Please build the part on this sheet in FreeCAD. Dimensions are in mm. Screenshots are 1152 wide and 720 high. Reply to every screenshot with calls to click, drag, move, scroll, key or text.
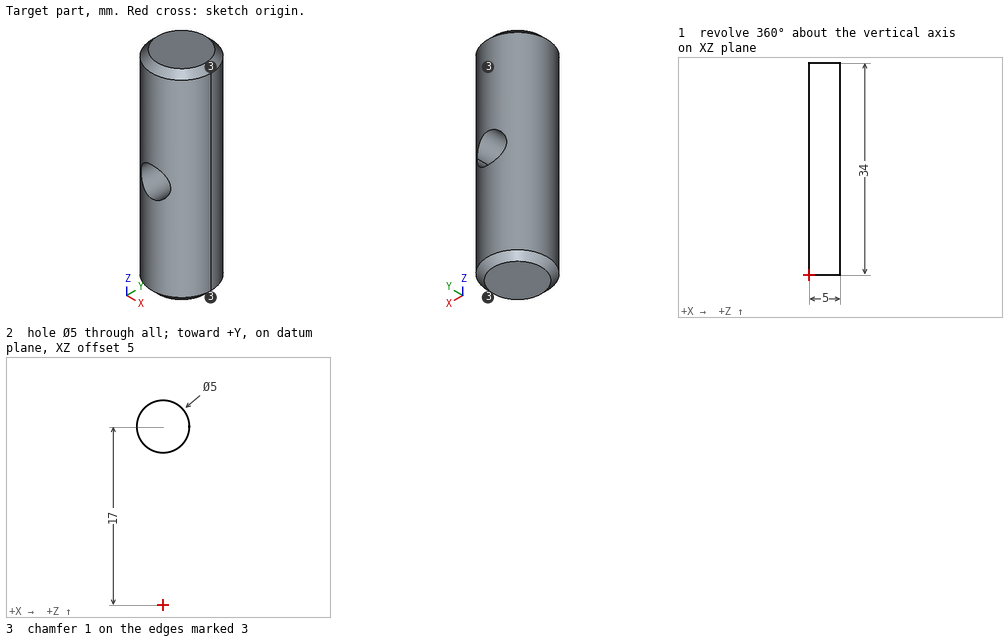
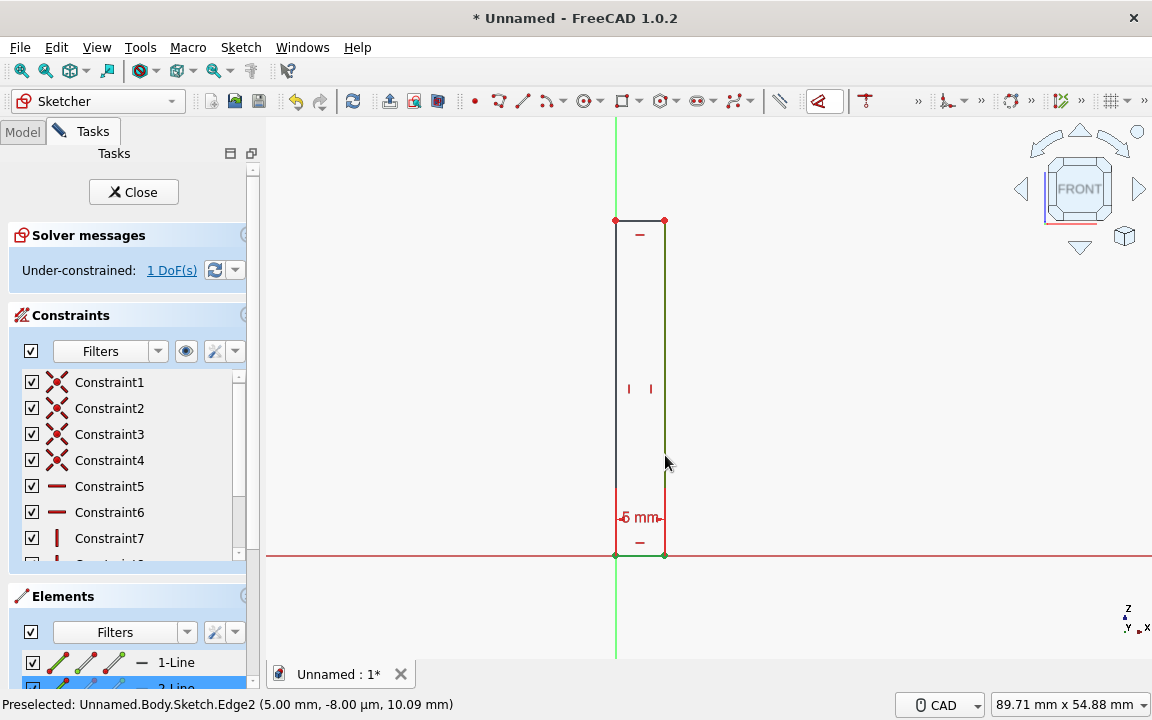
key(i)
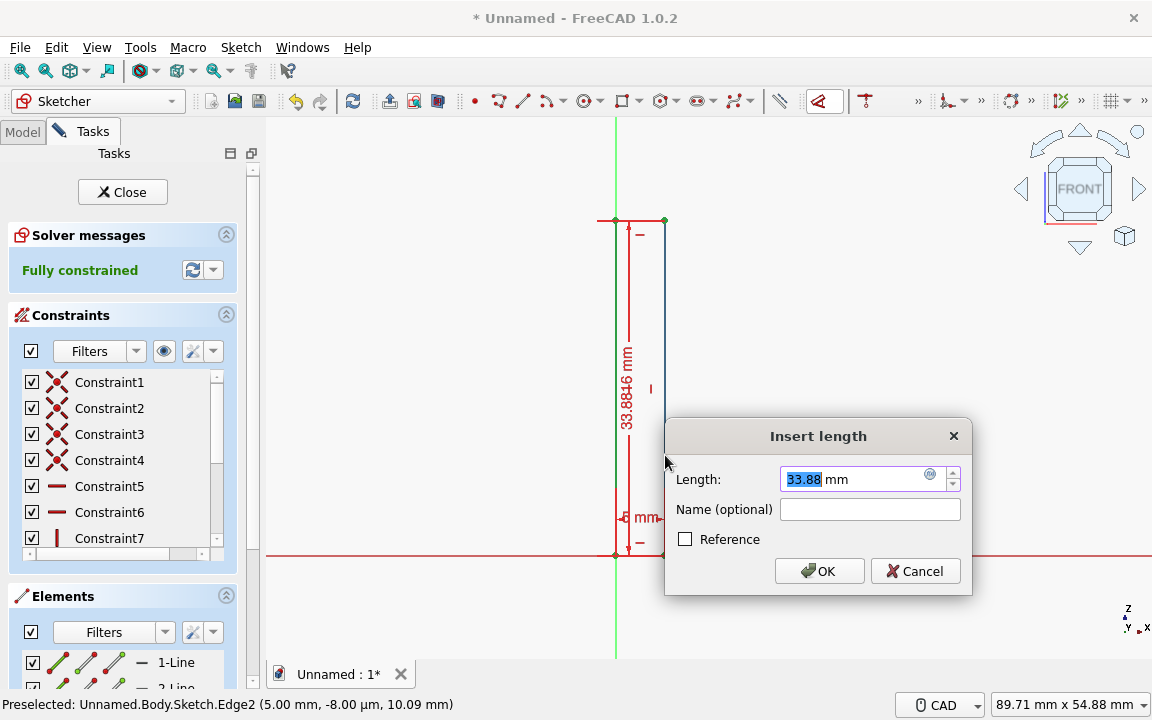
text(34)
key(Return)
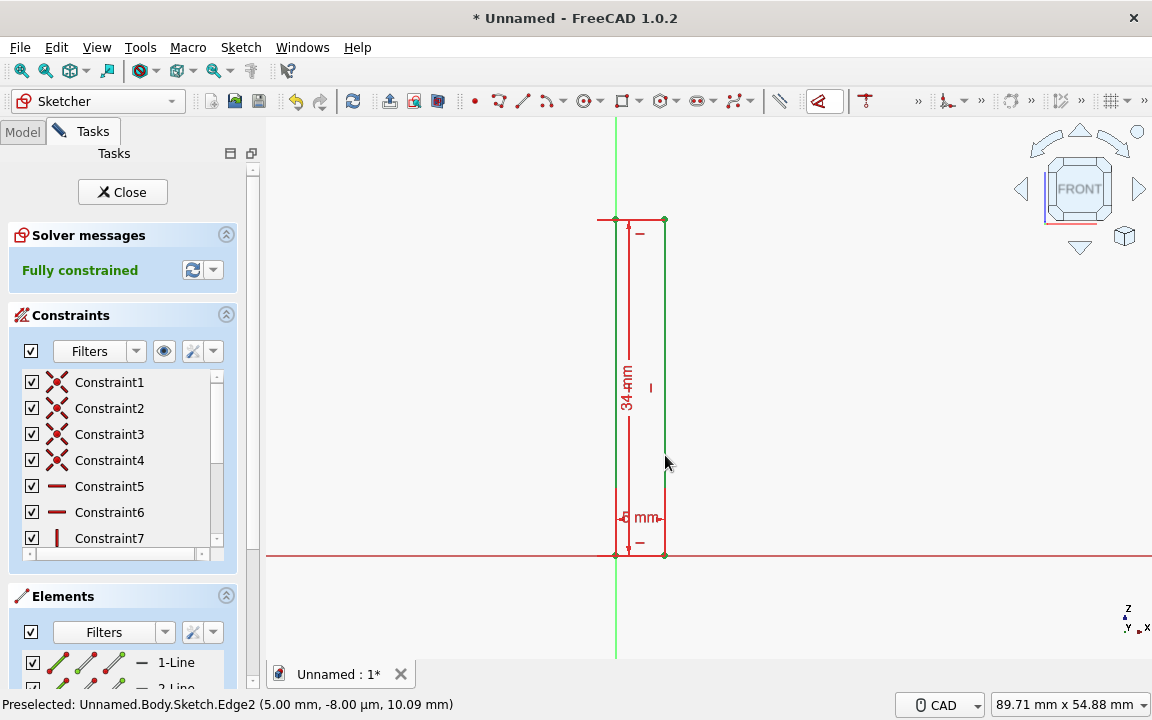
click(123, 192)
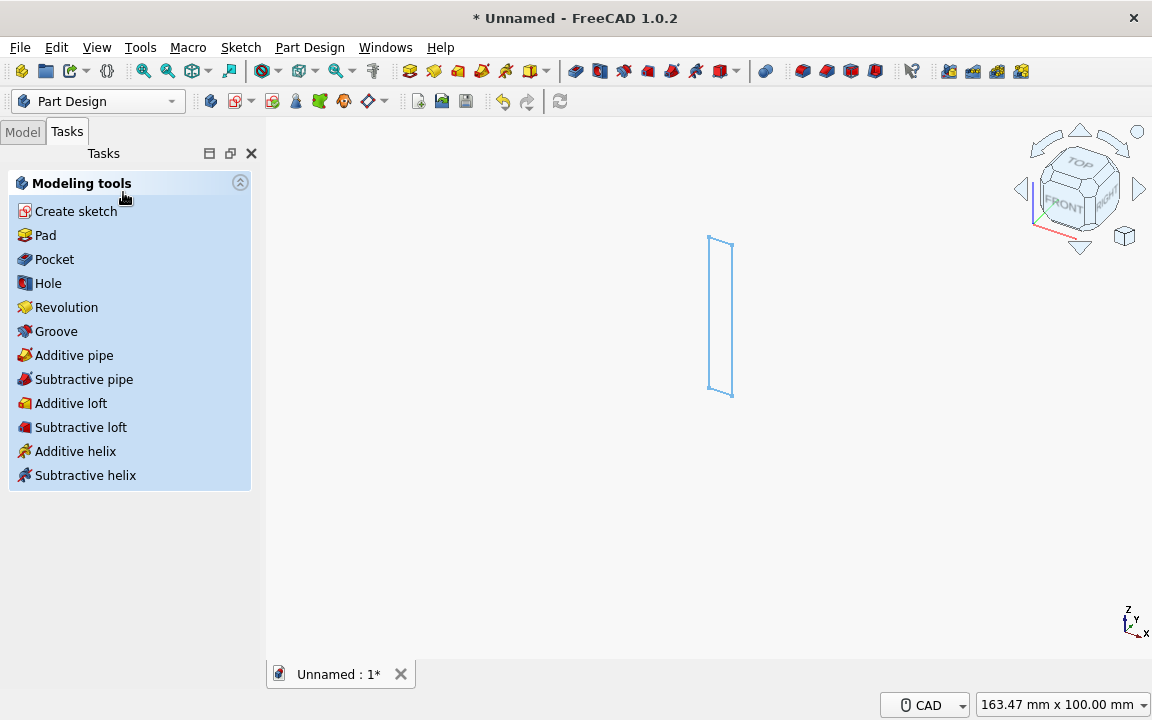
click(434, 72)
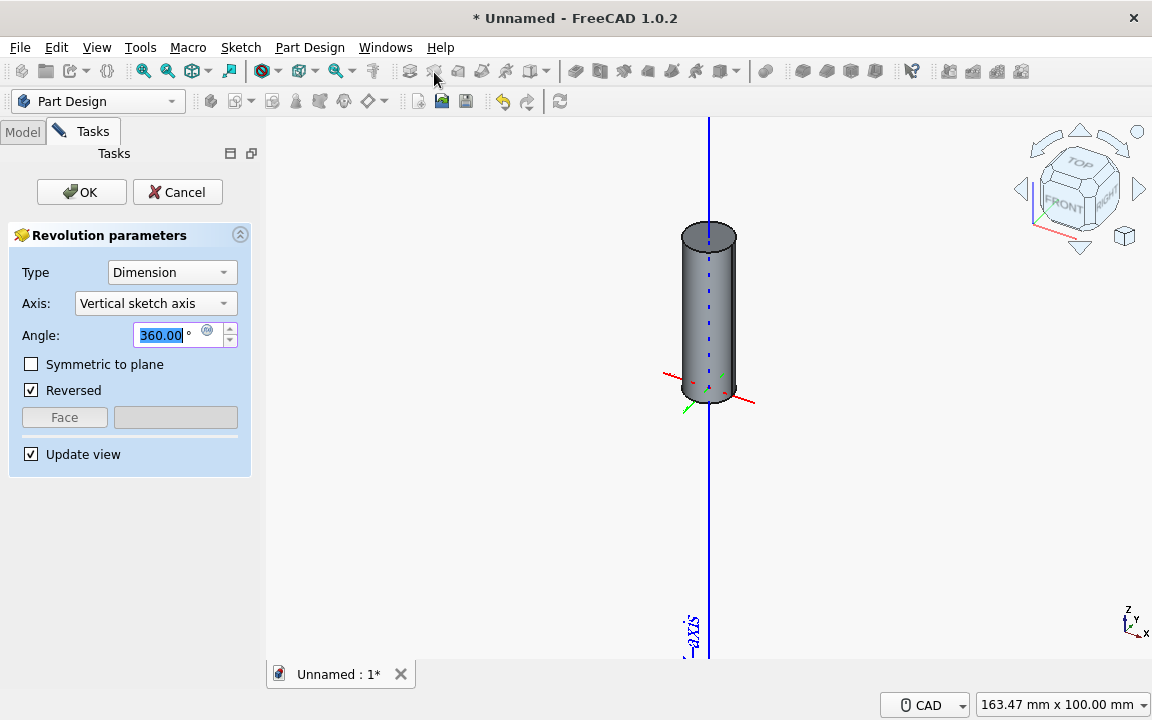
click(82, 192)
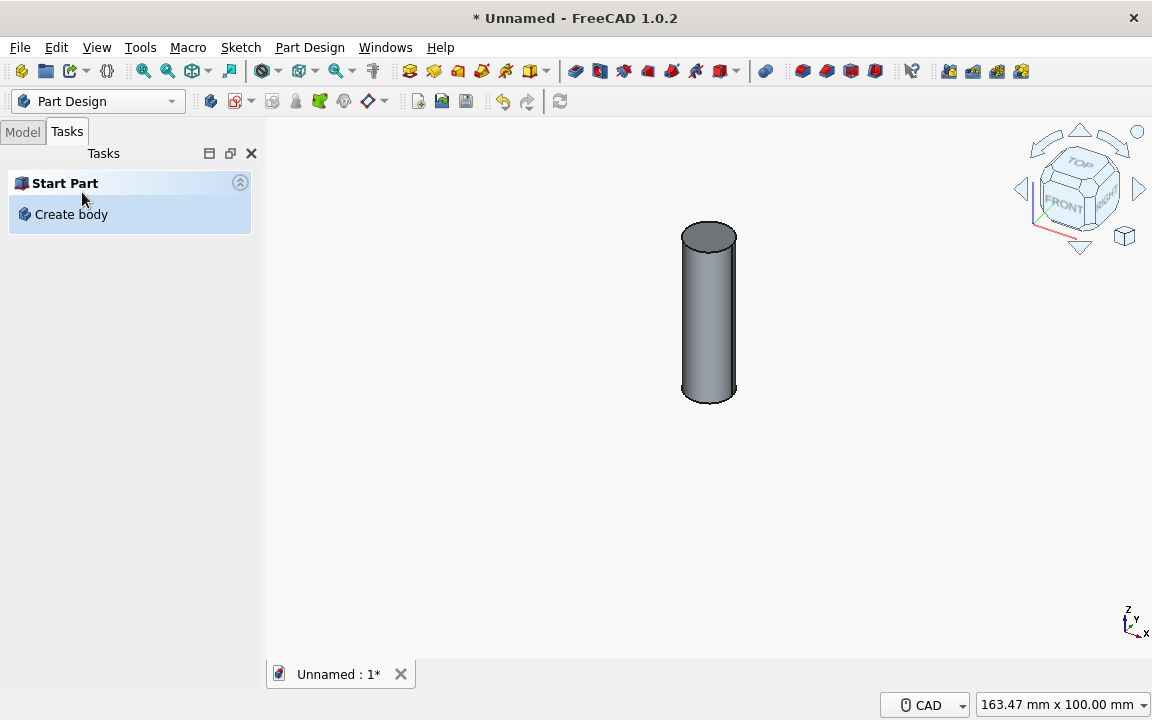
click(144, 72)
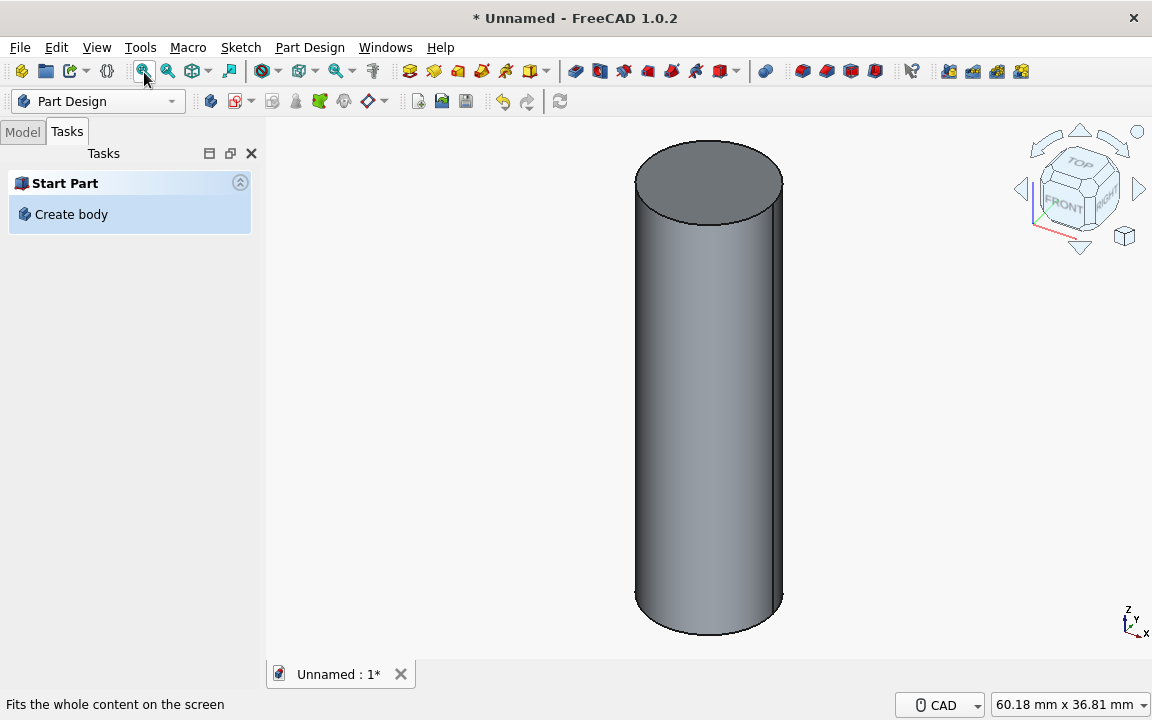
click(23, 131)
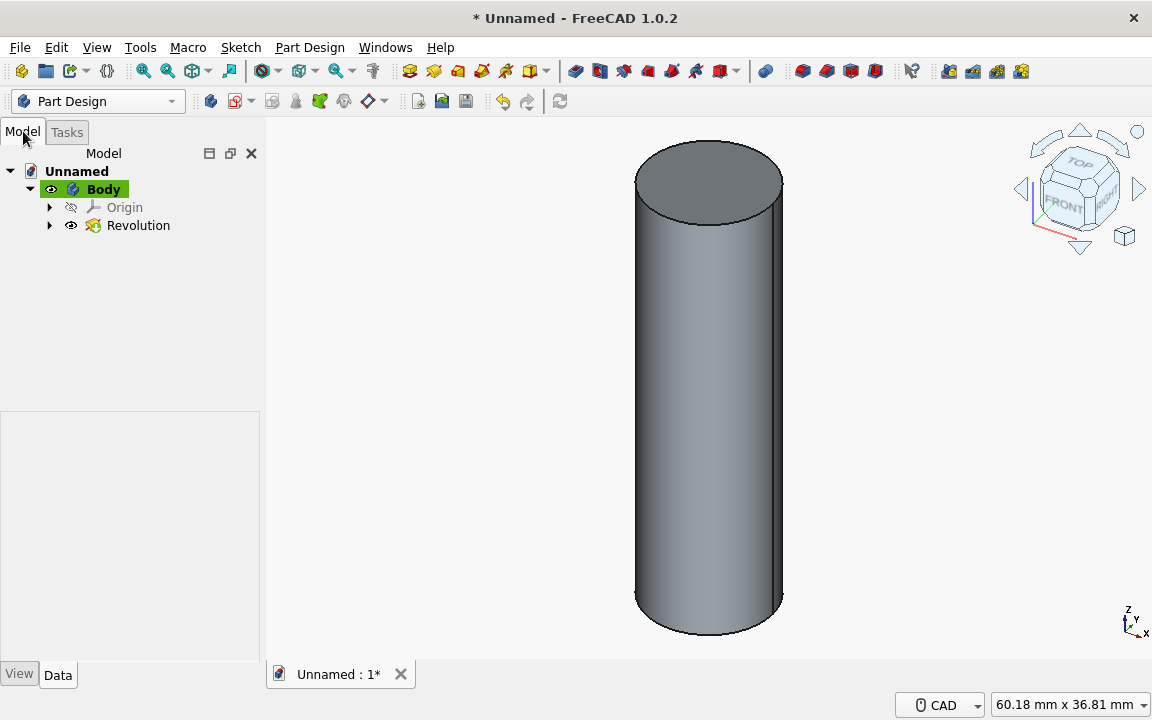
click(50, 207)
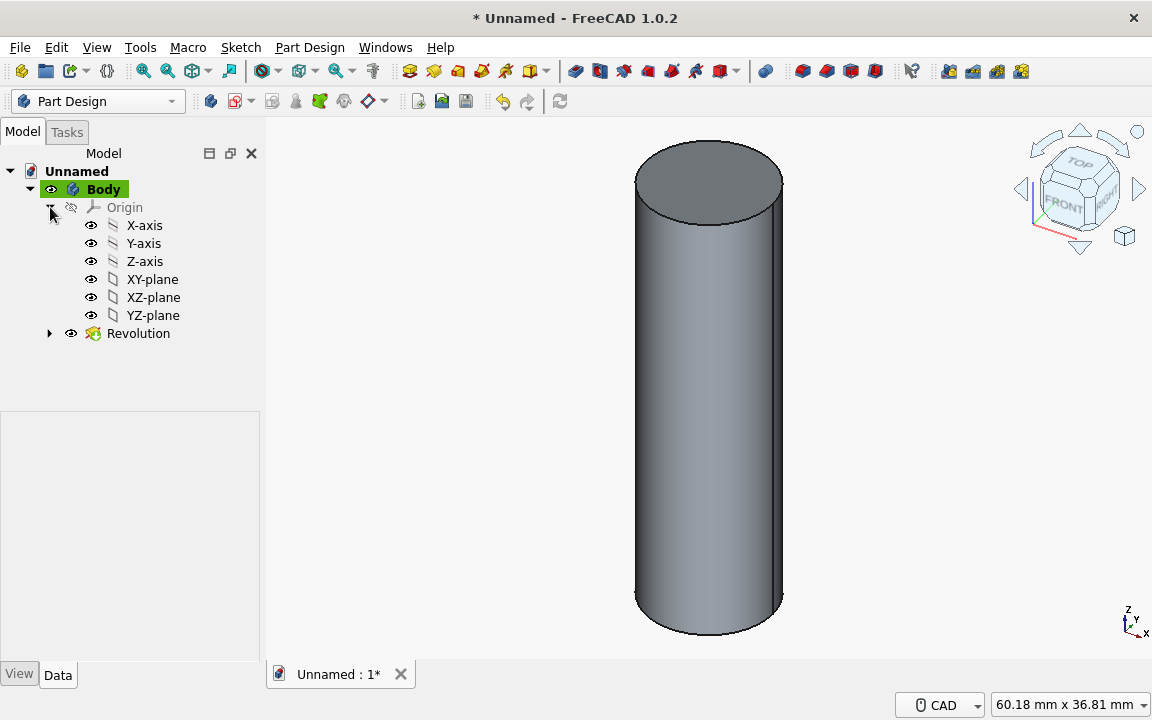
click(136, 297)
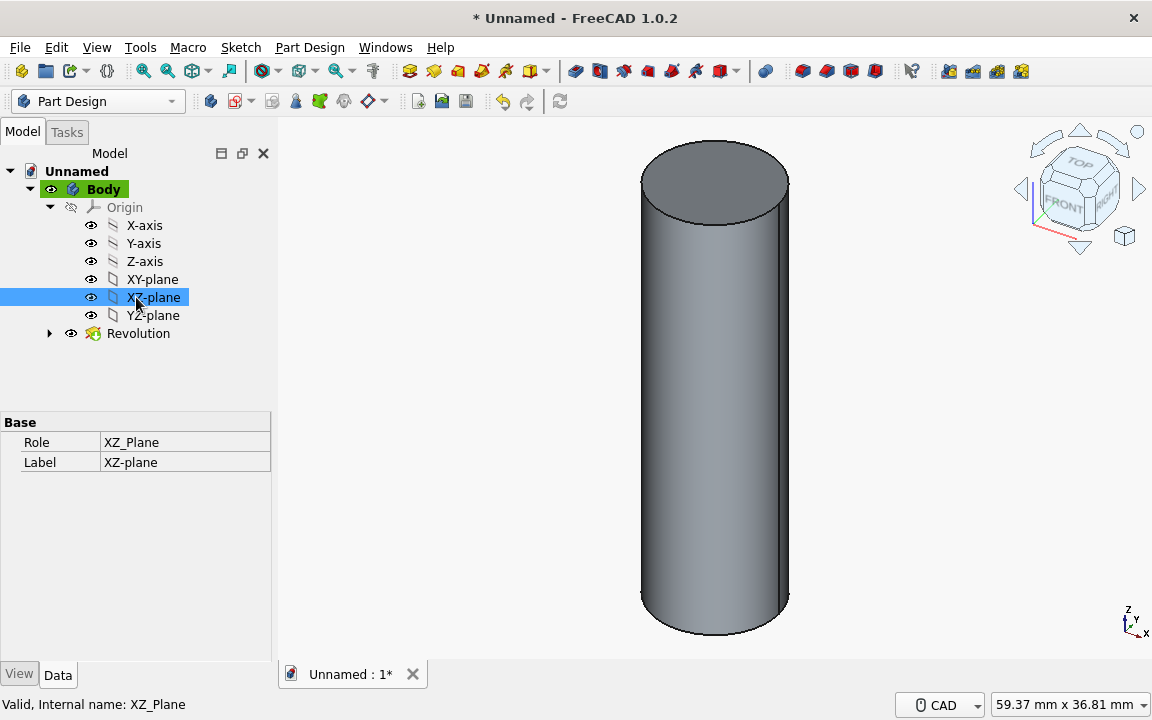
click(368, 102)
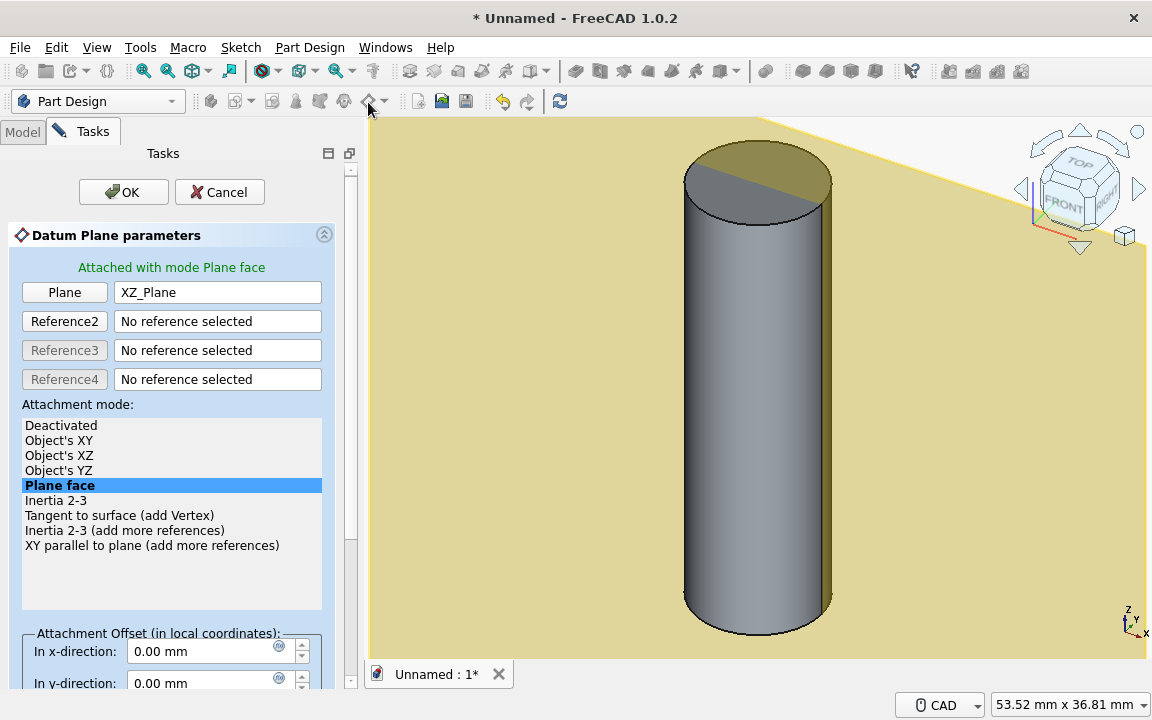
scroll(351, 426, down, 2)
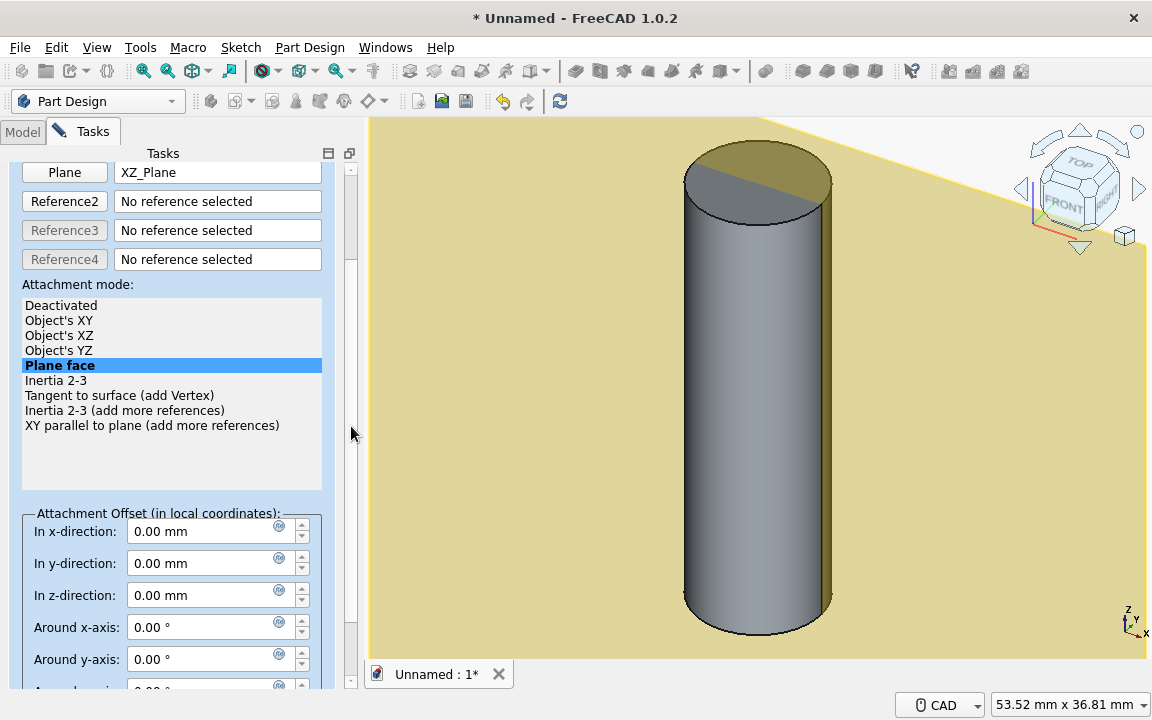
triple_click(210, 595)